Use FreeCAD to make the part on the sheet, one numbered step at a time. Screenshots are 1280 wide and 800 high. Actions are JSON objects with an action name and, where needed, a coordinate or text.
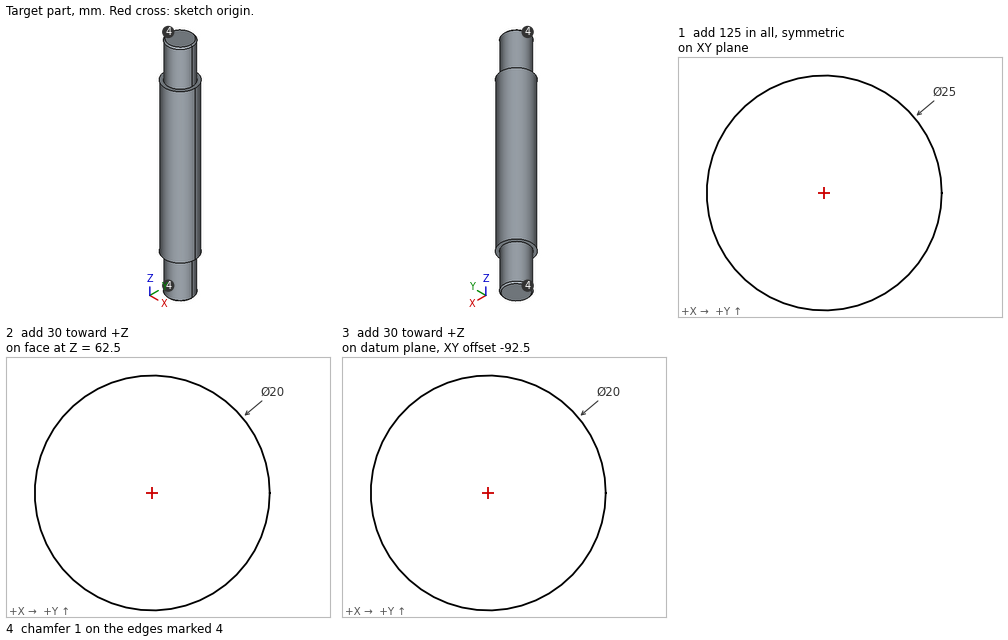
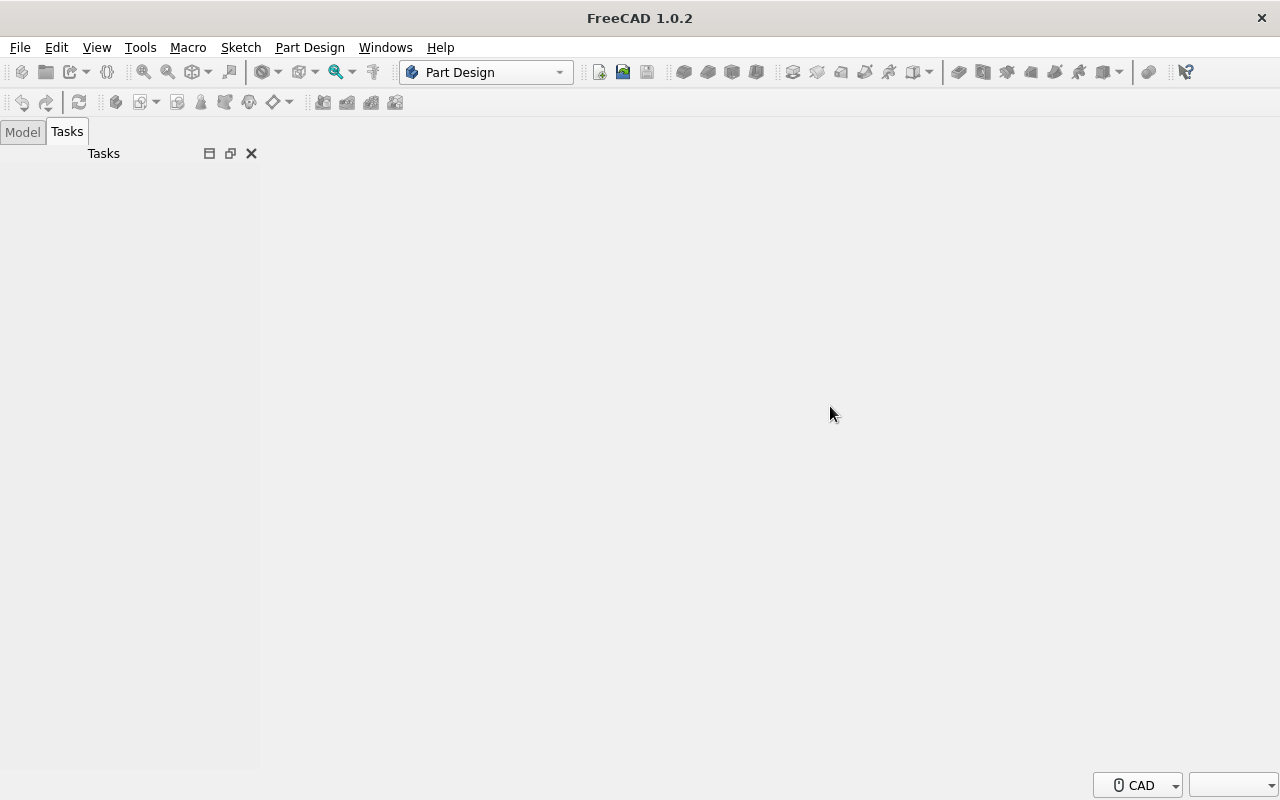
{"action": "key", "text": "ctrl+n"}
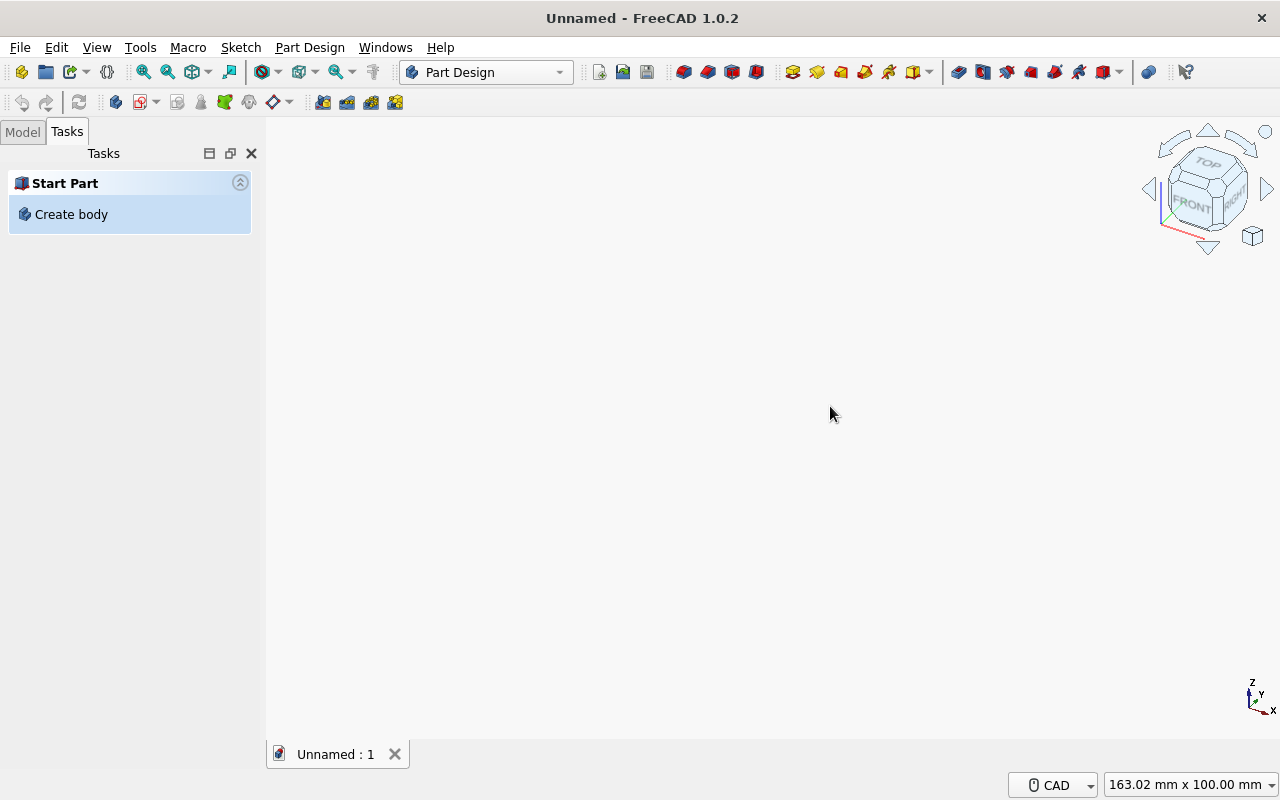
{"action": "left_click", "coordinate": [140, 102]}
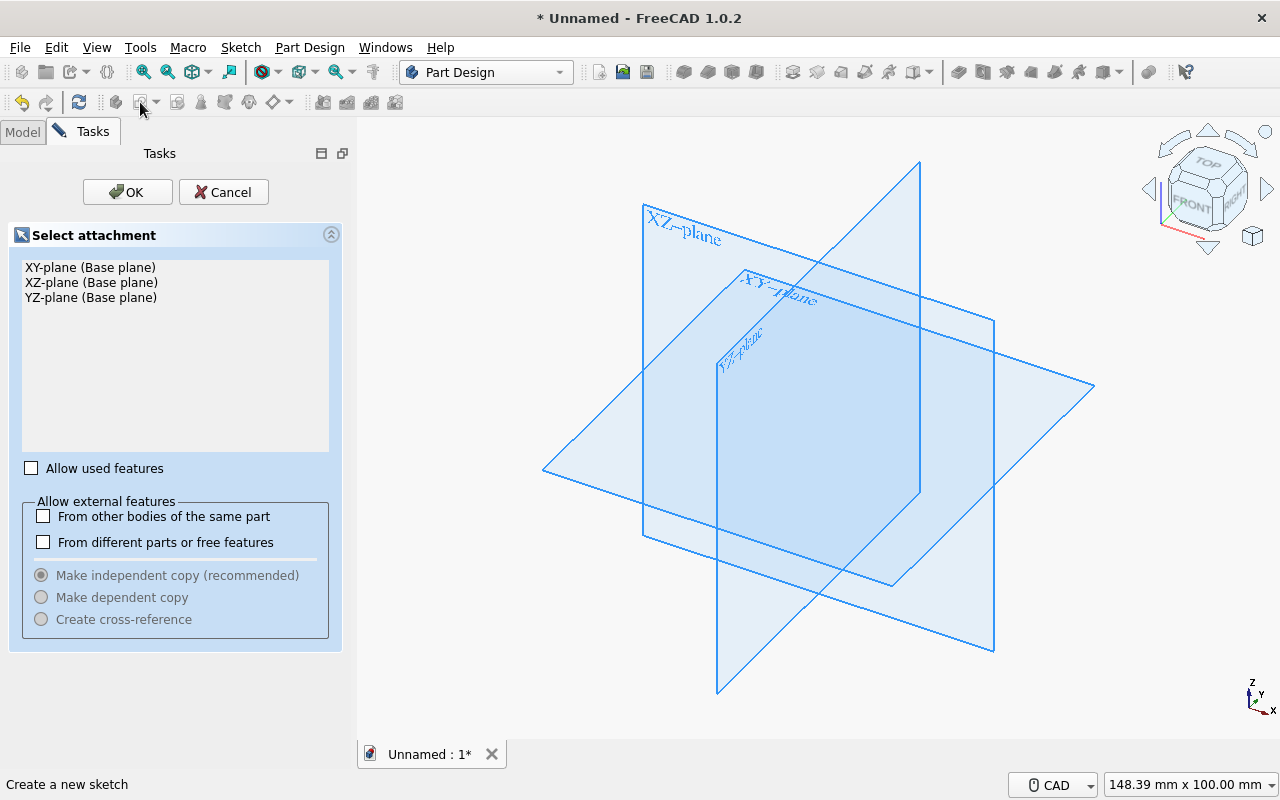
{"action": "left_click", "coordinate": [82, 268]}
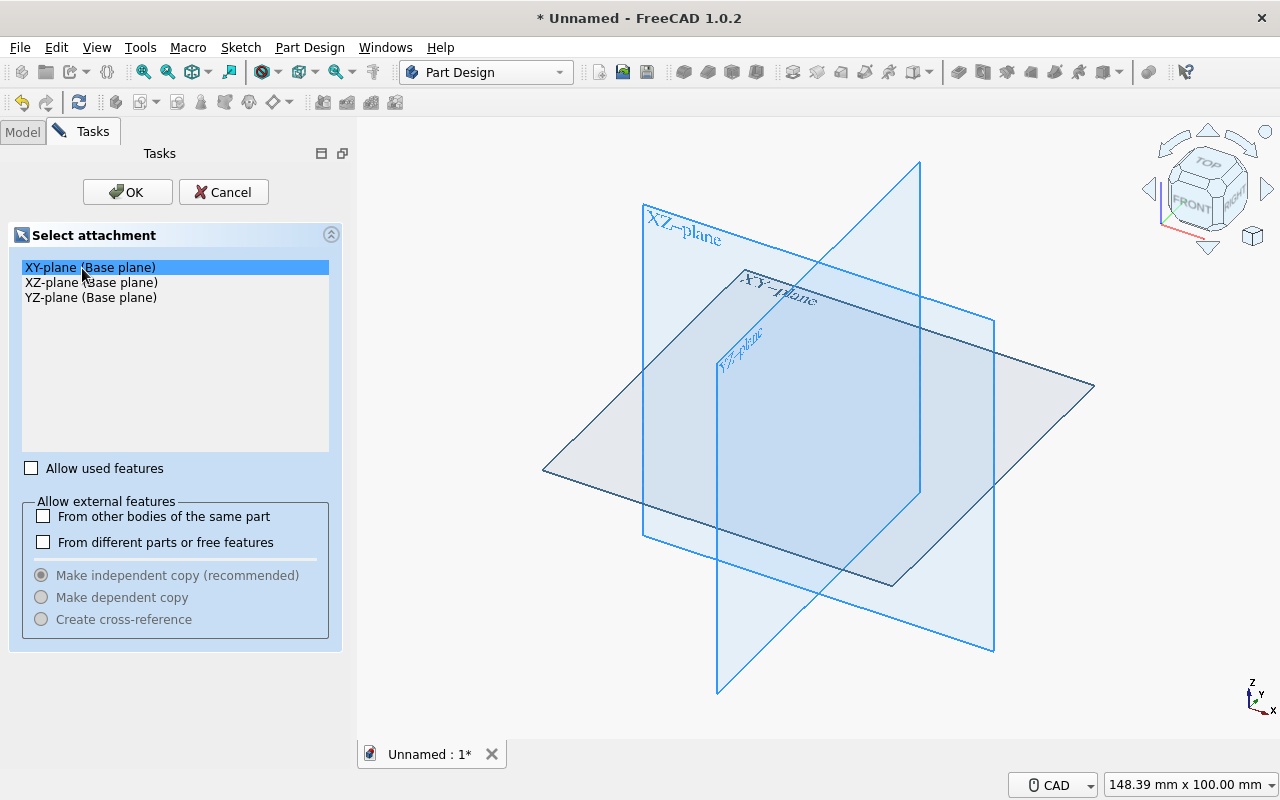
{"action": "left_click", "coordinate": [128, 192]}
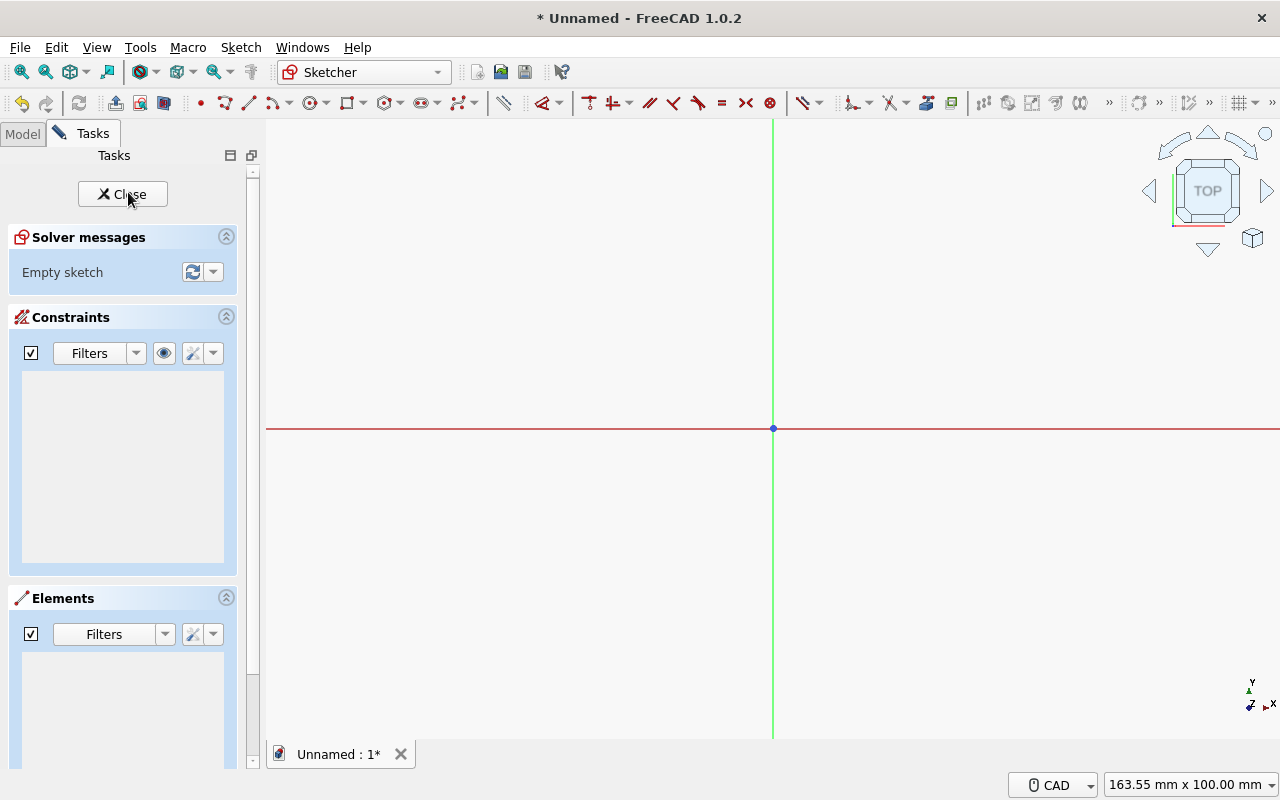
{"action": "scroll", "coordinate": [813, 429], "scroll_direction": "up", "scroll_amount": 5}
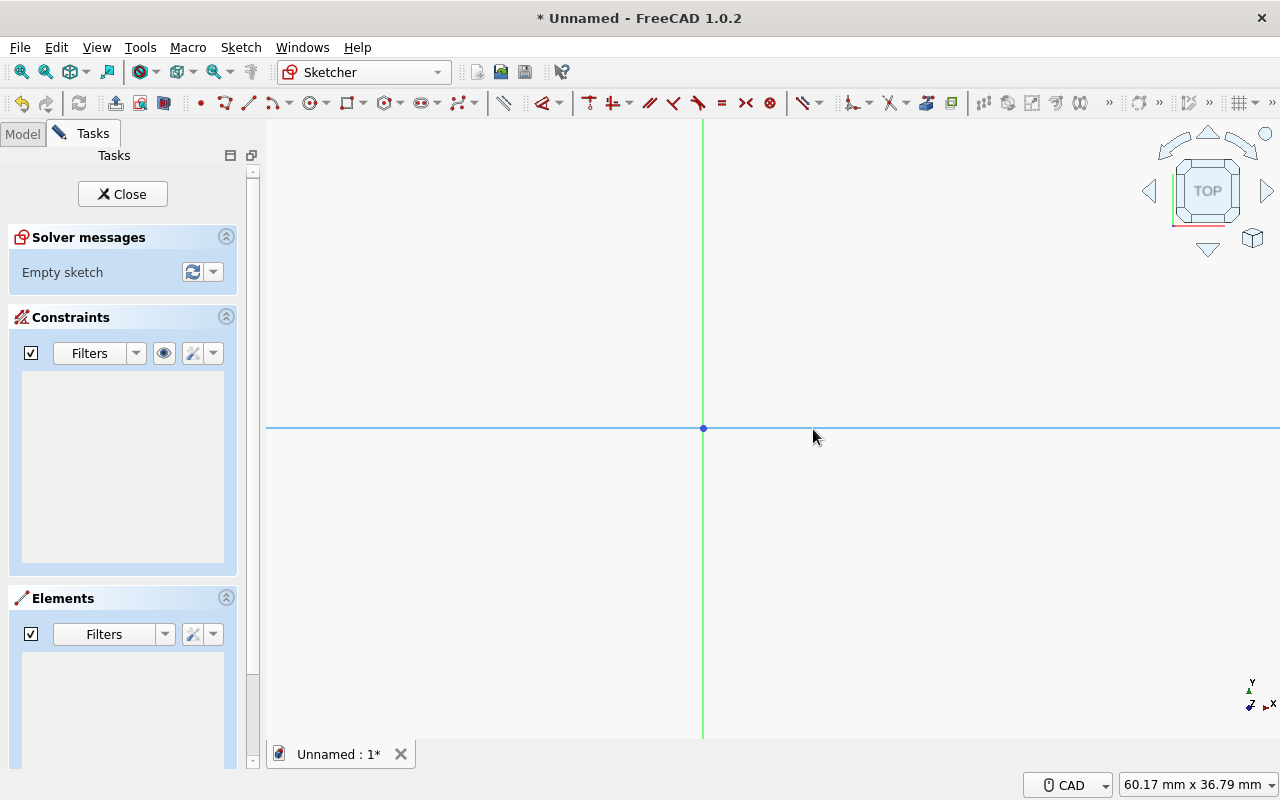
{"action": "key", "text": "g c"}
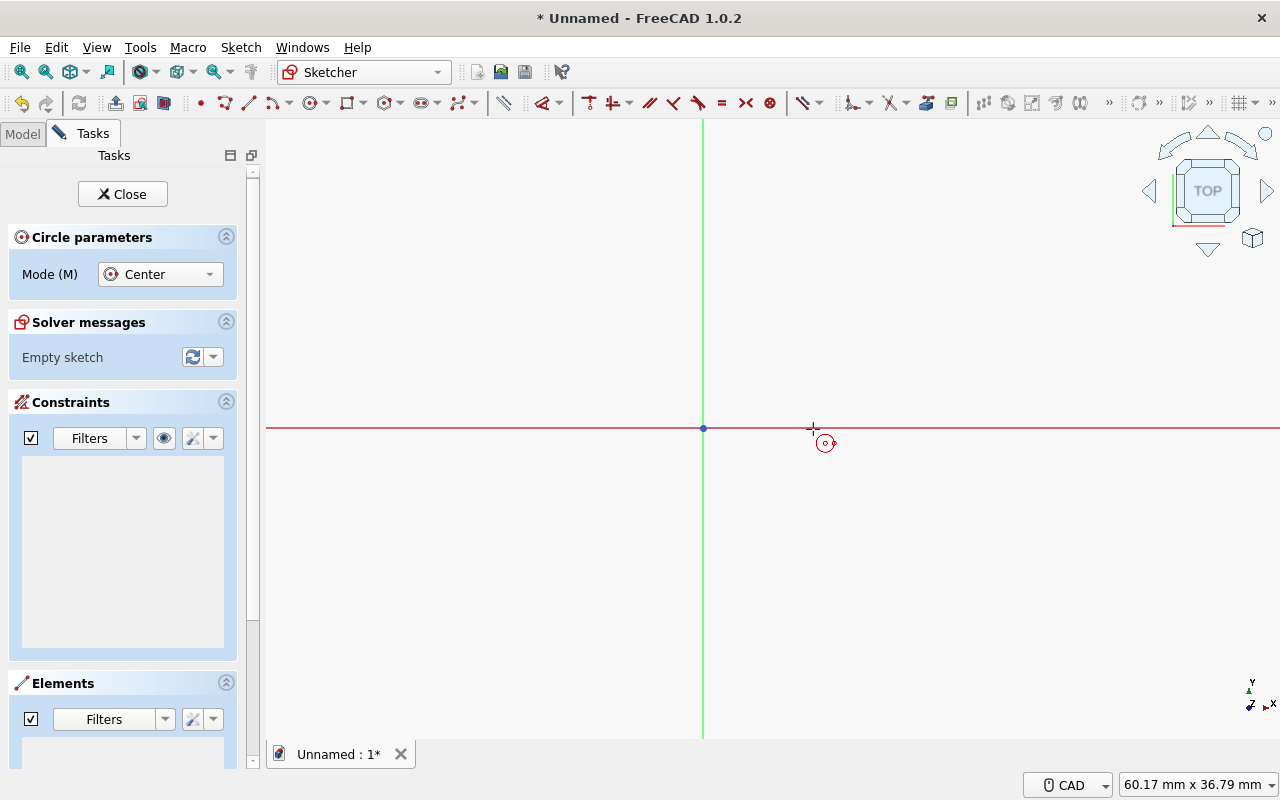
{"action": "left_click", "coordinate": [703, 428]}
{"action": "left_click", "coordinate": [852, 279]}
{"action": "key", "text": "Escape"}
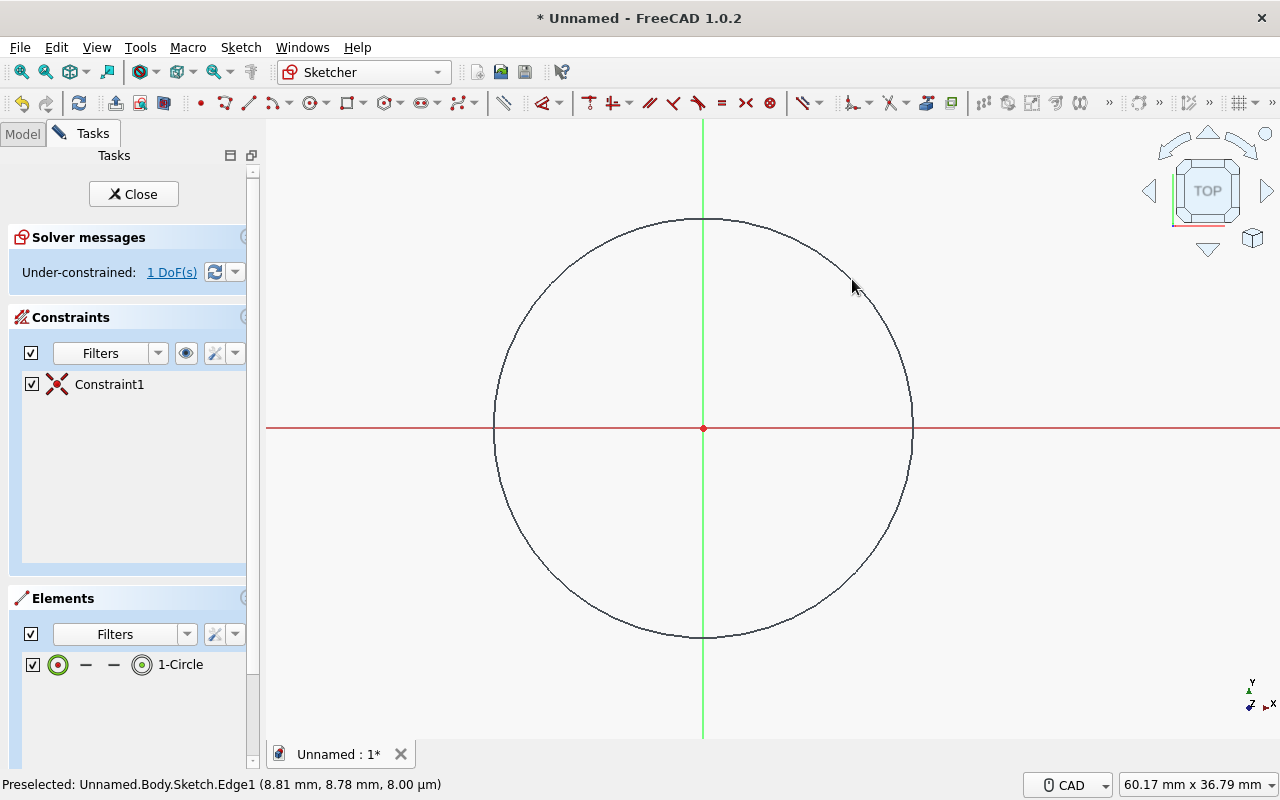
{"action": "left_click", "coordinate": [851, 279]}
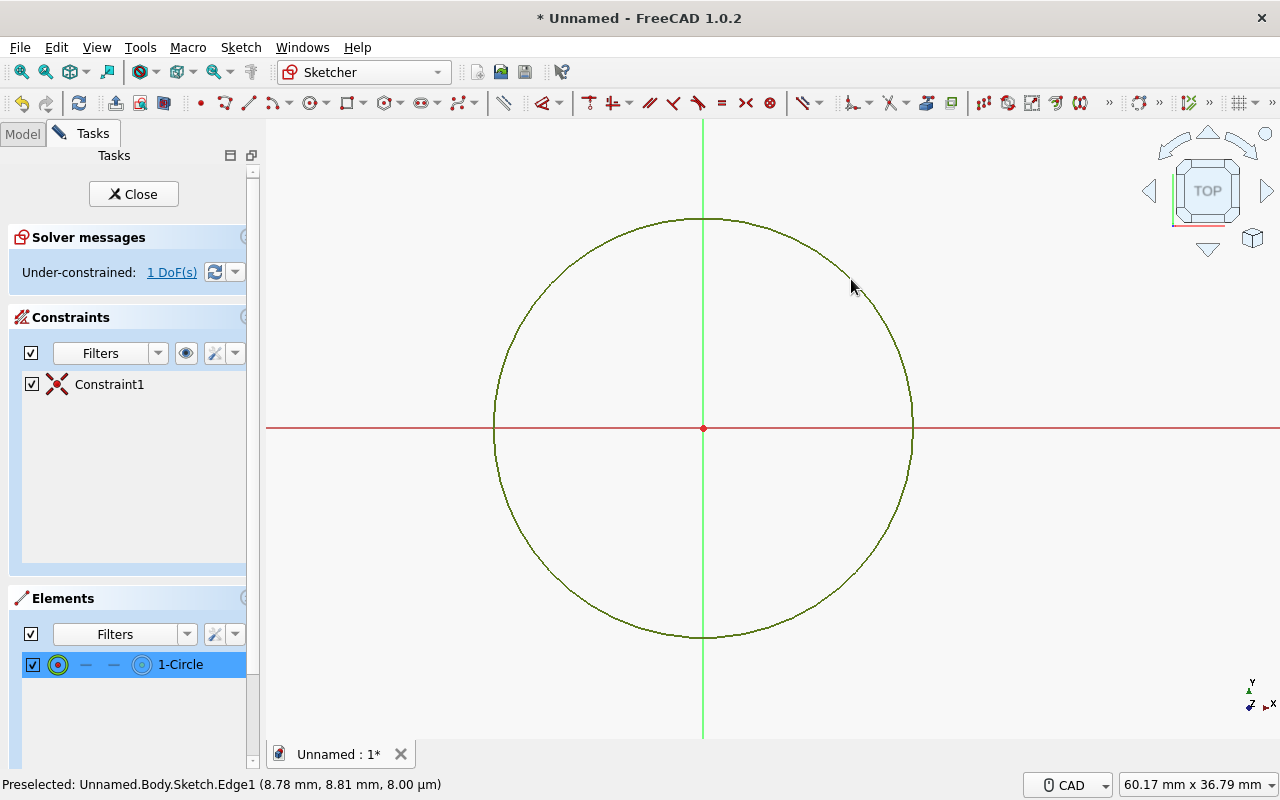
{"action": "left_click", "coordinate": [562, 104]}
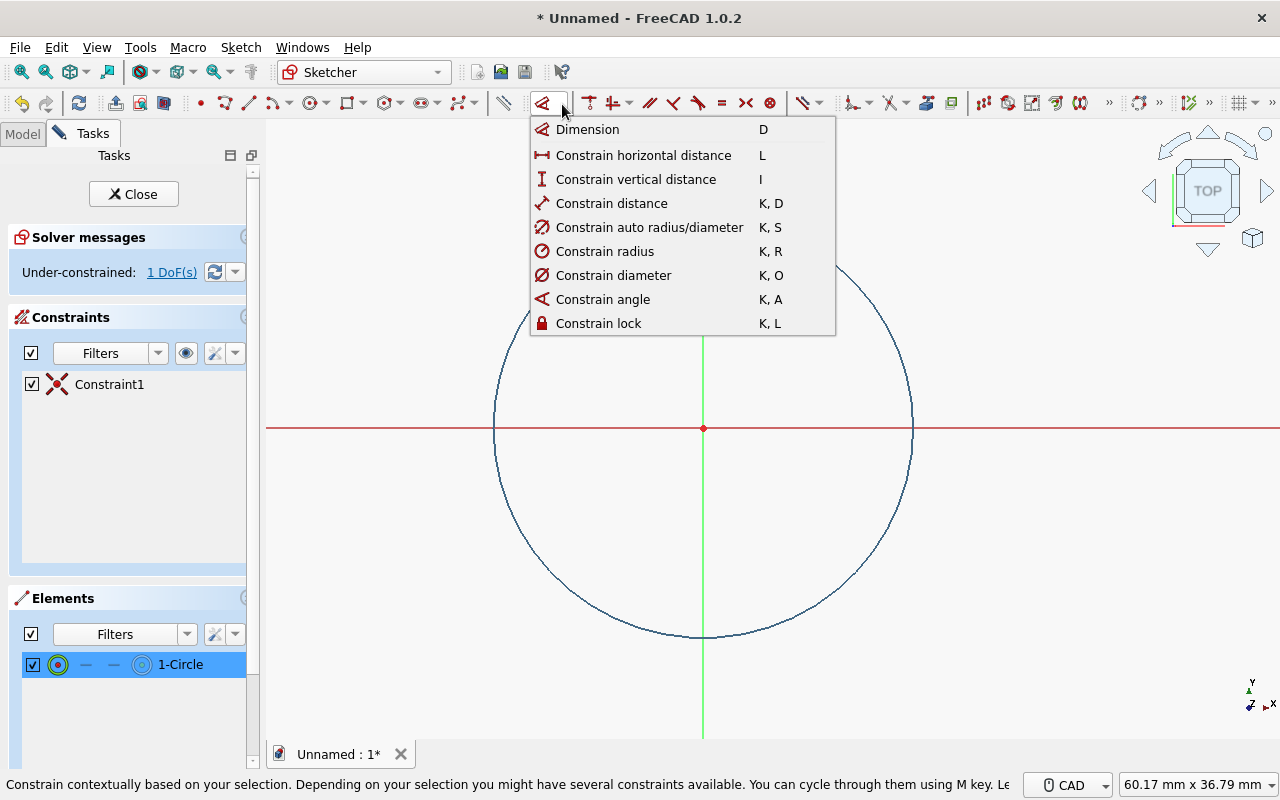
{"action": "left_click", "coordinate": [683, 275]}